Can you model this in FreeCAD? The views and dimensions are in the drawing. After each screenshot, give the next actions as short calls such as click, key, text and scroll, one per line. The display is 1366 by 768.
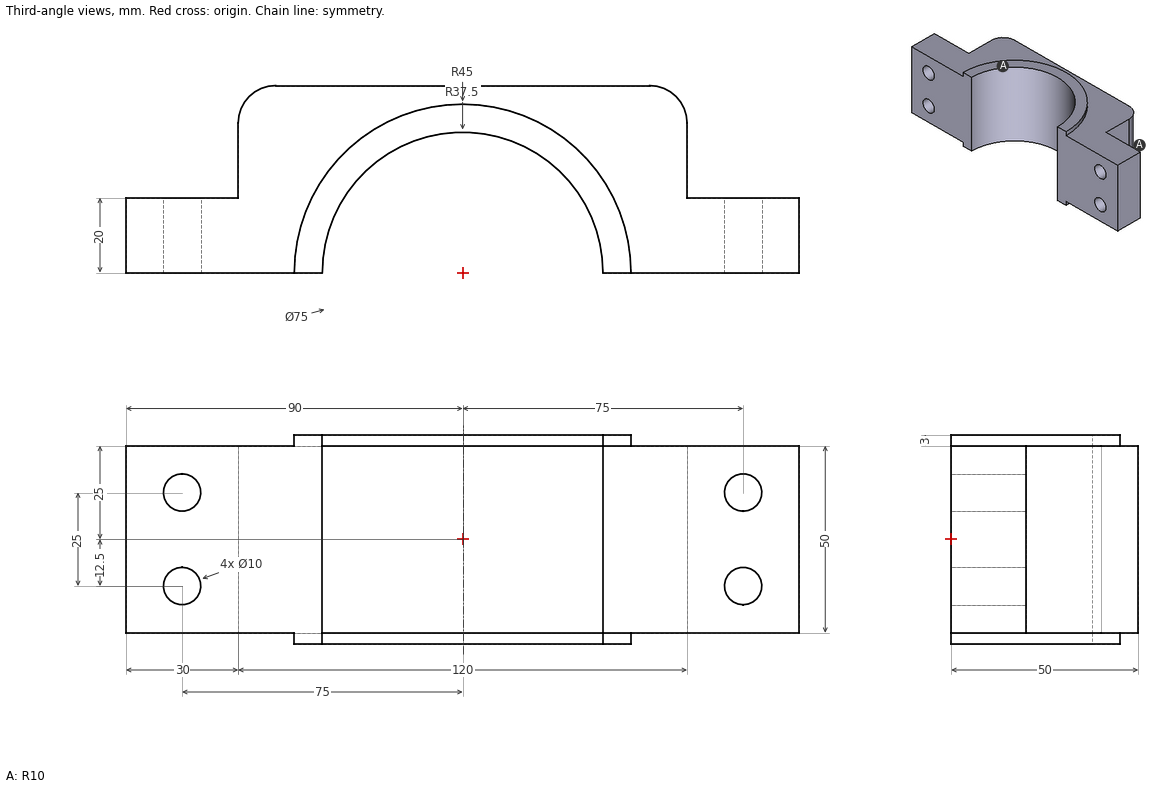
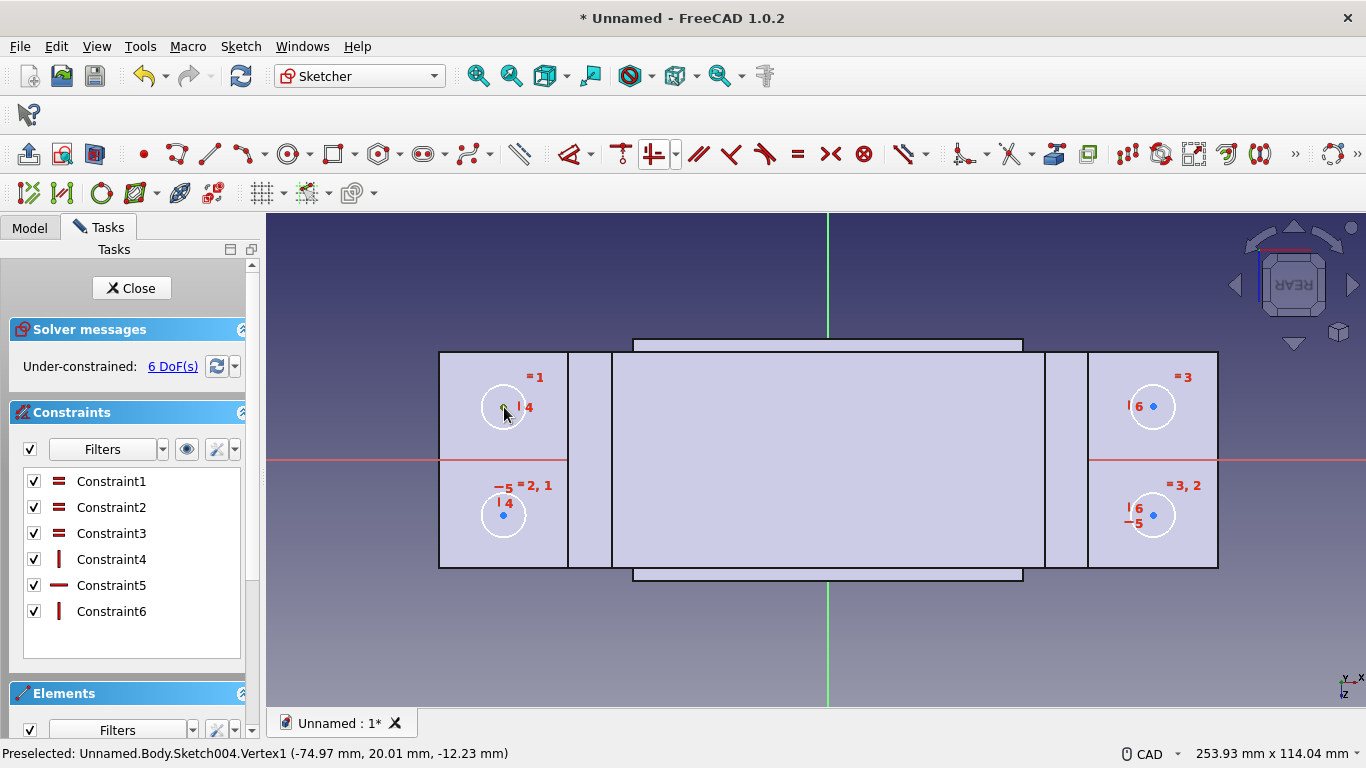
click(1153, 407)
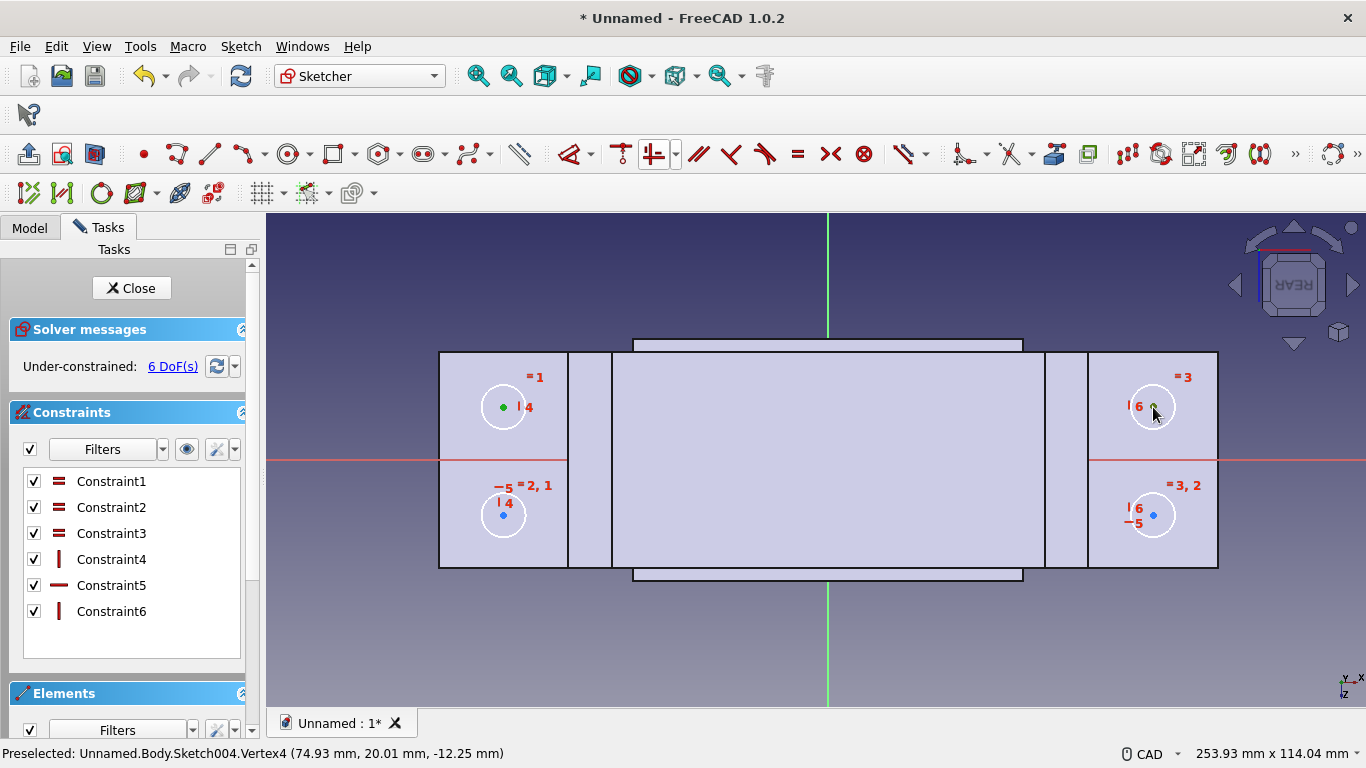
key(h)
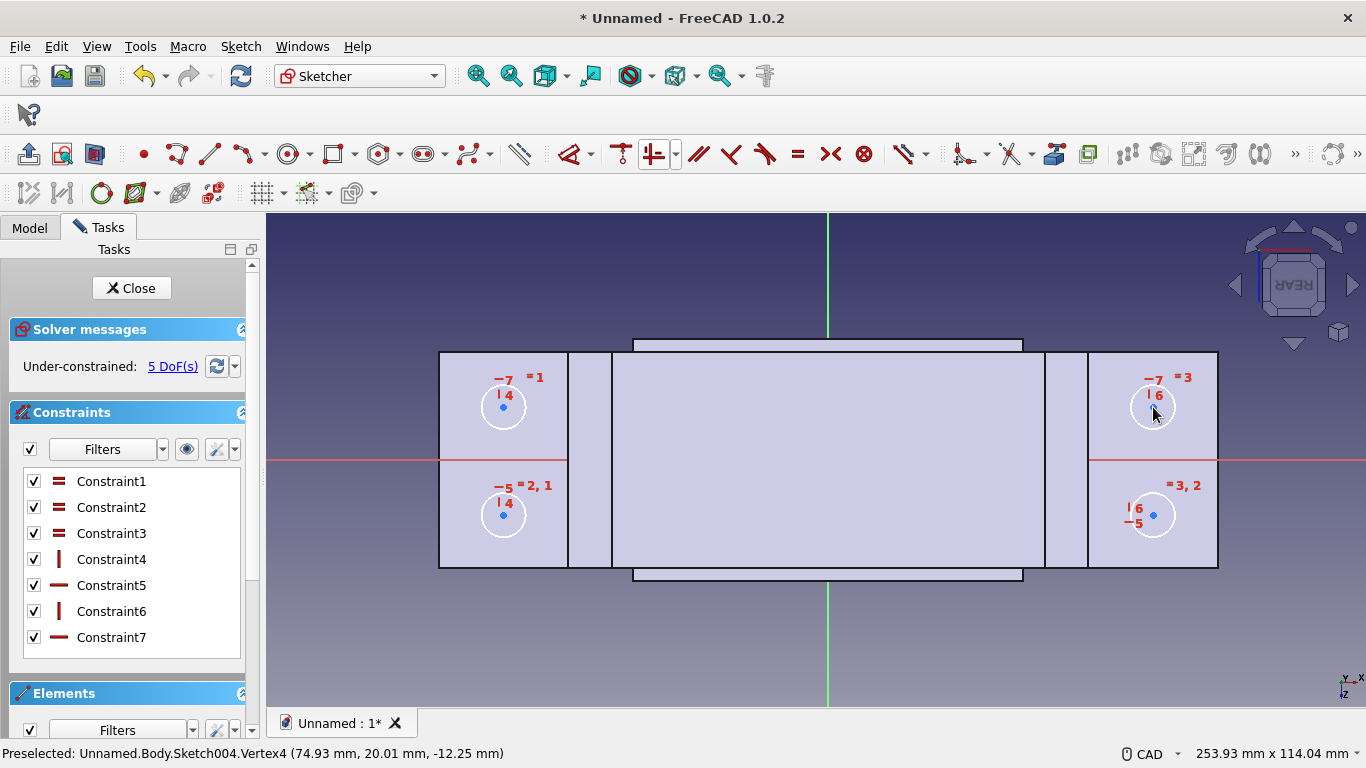
click(519, 391)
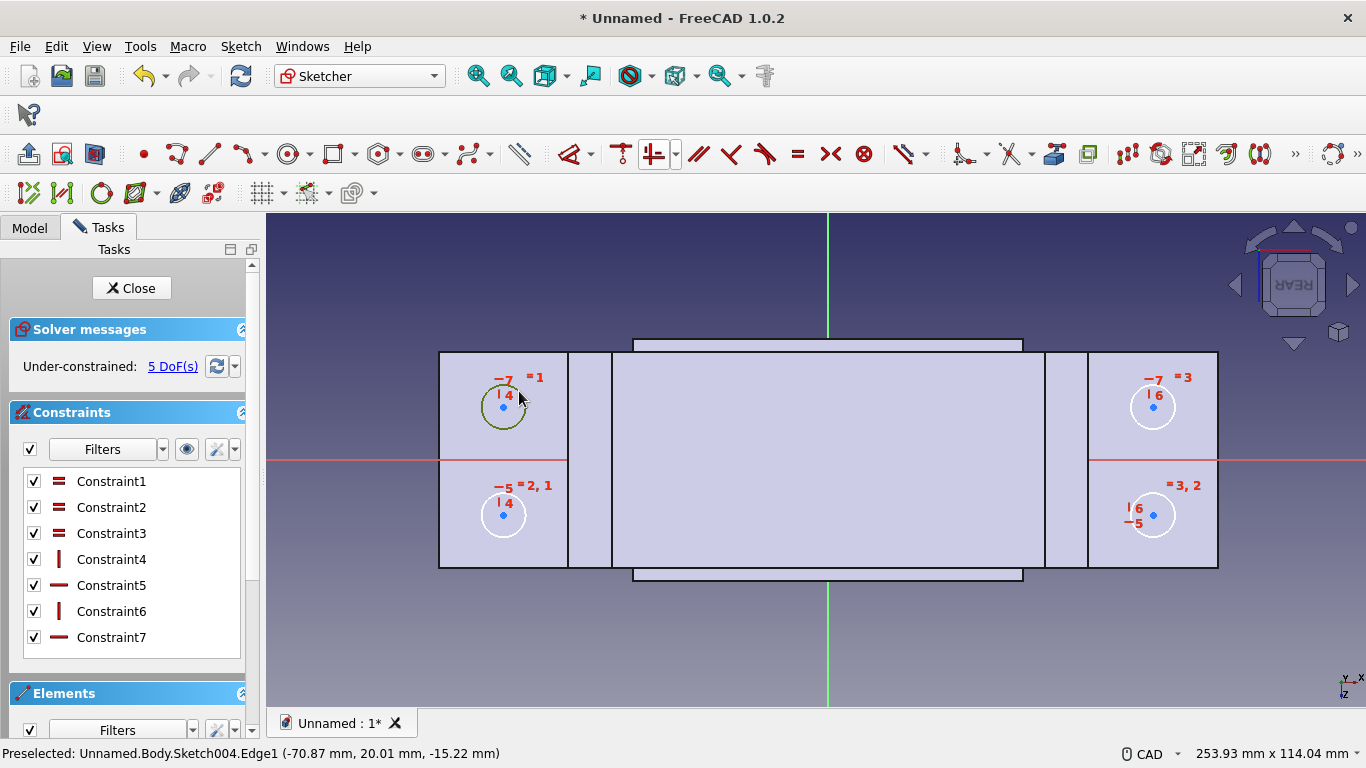
key(k)
key(o)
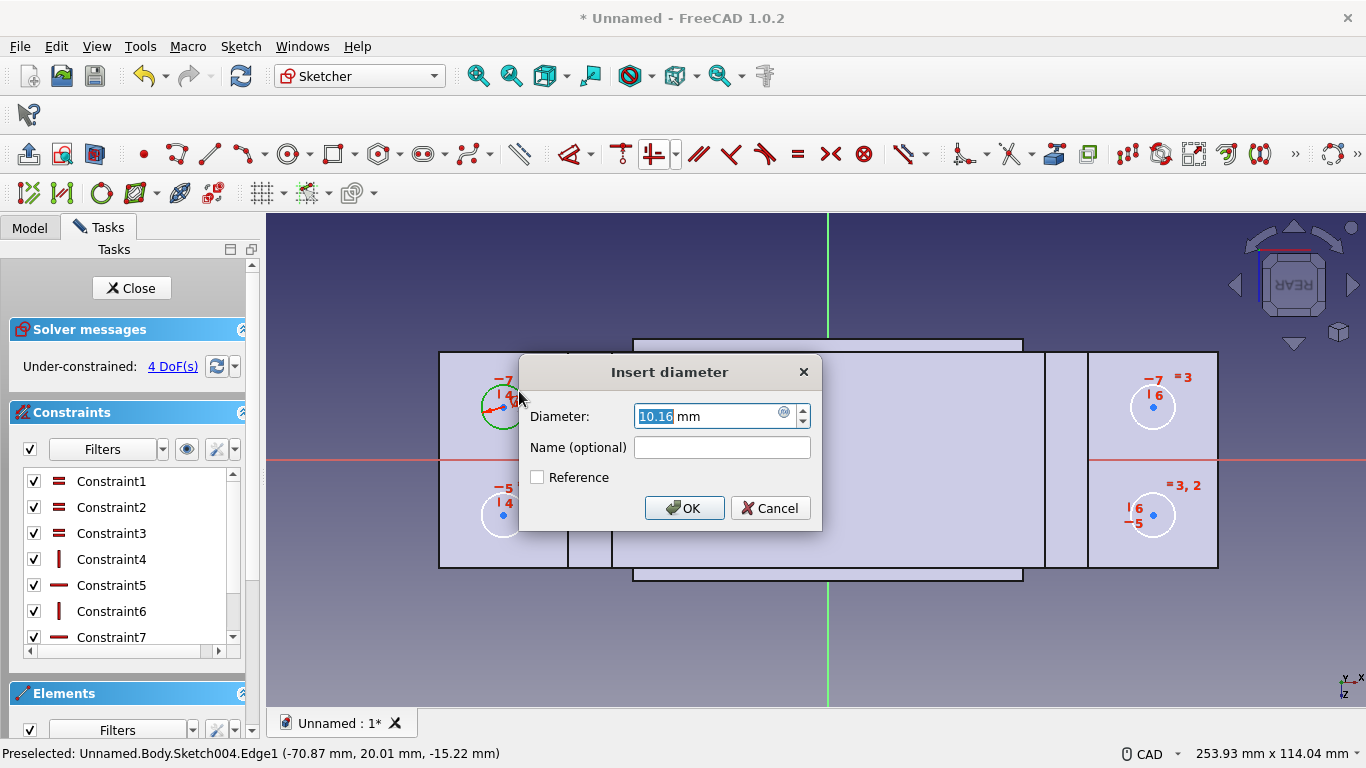
text(10)
key(Return)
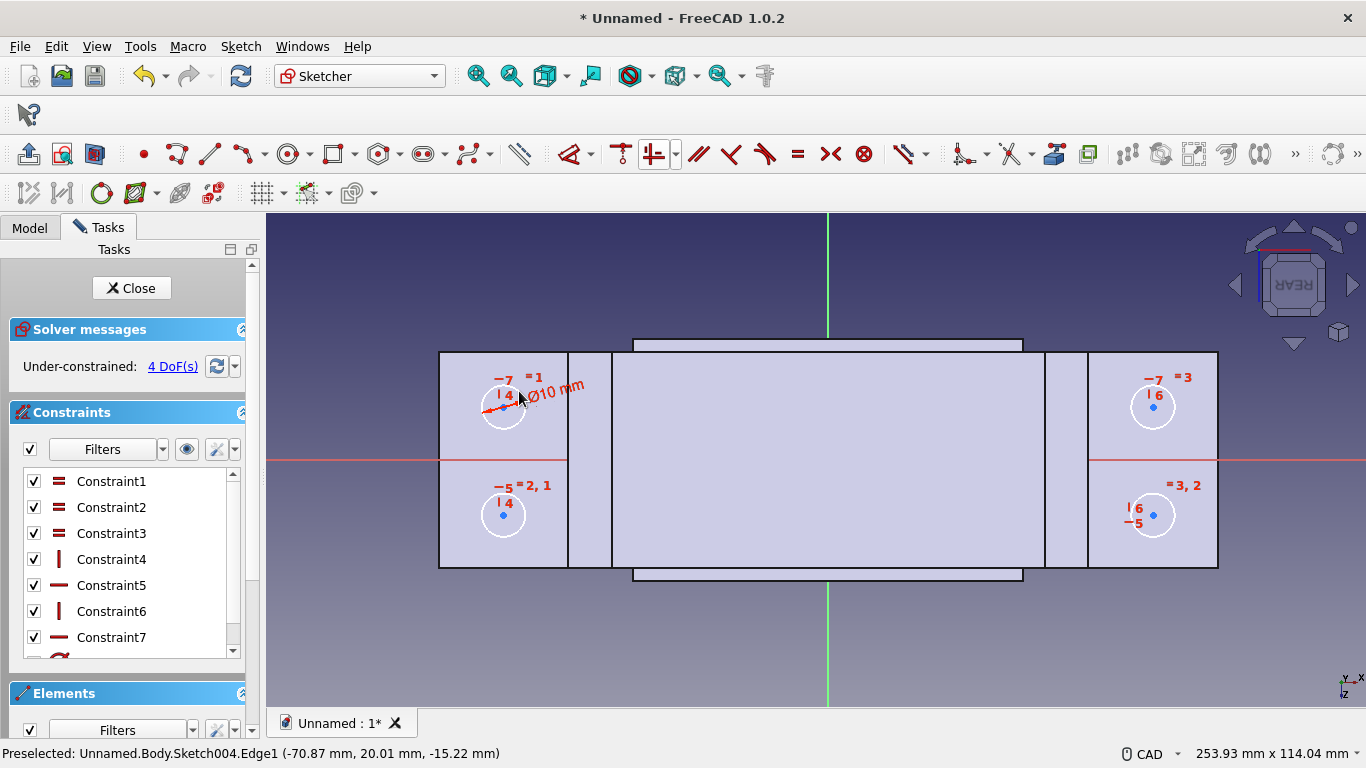
click(504, 407)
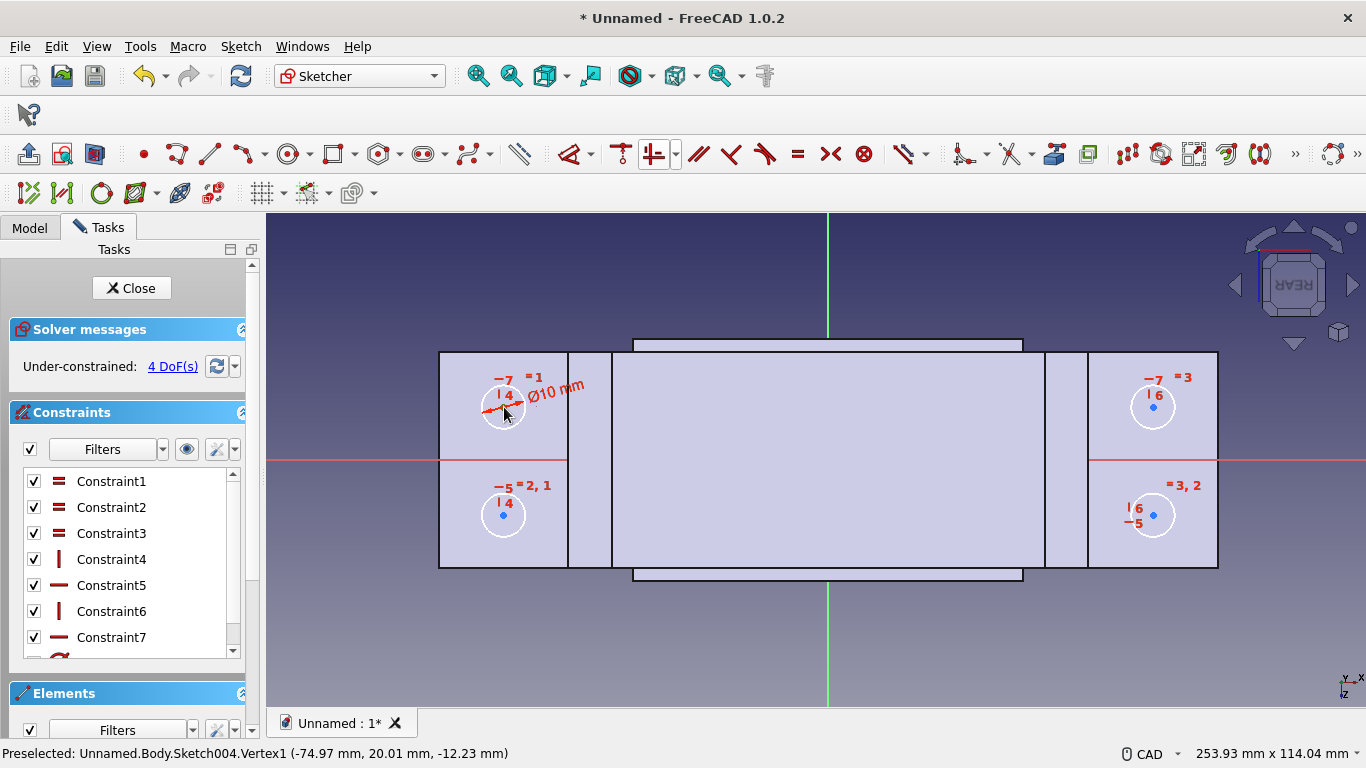
click(590, 154)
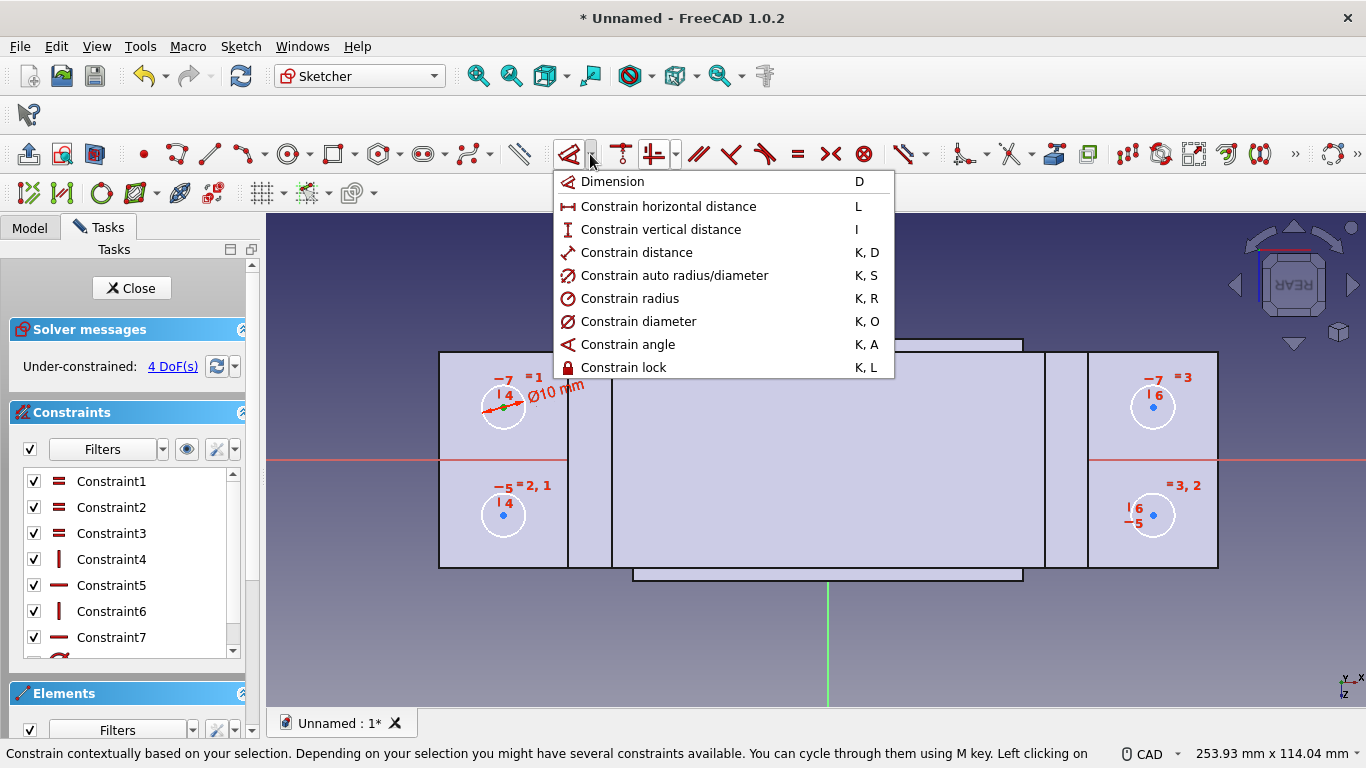
click(724, 206)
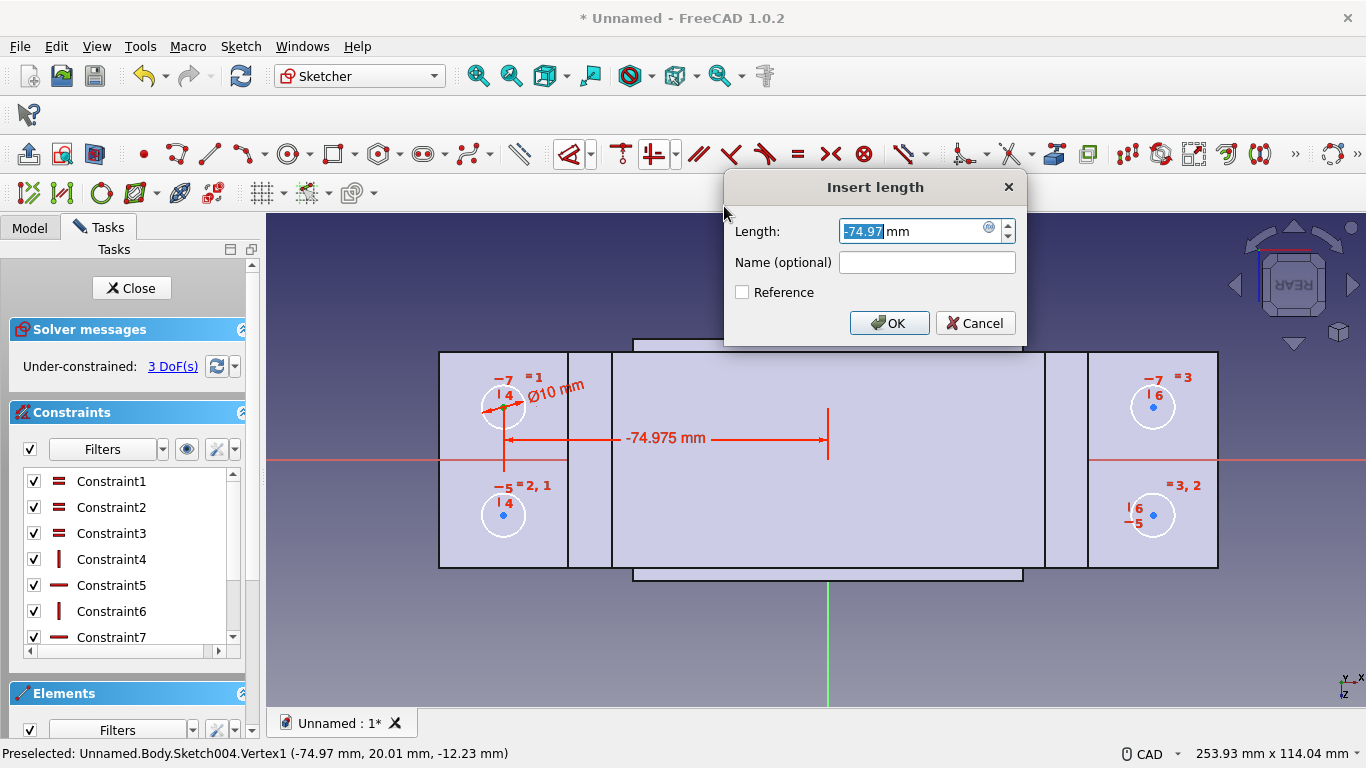
text(-75)
key(Return)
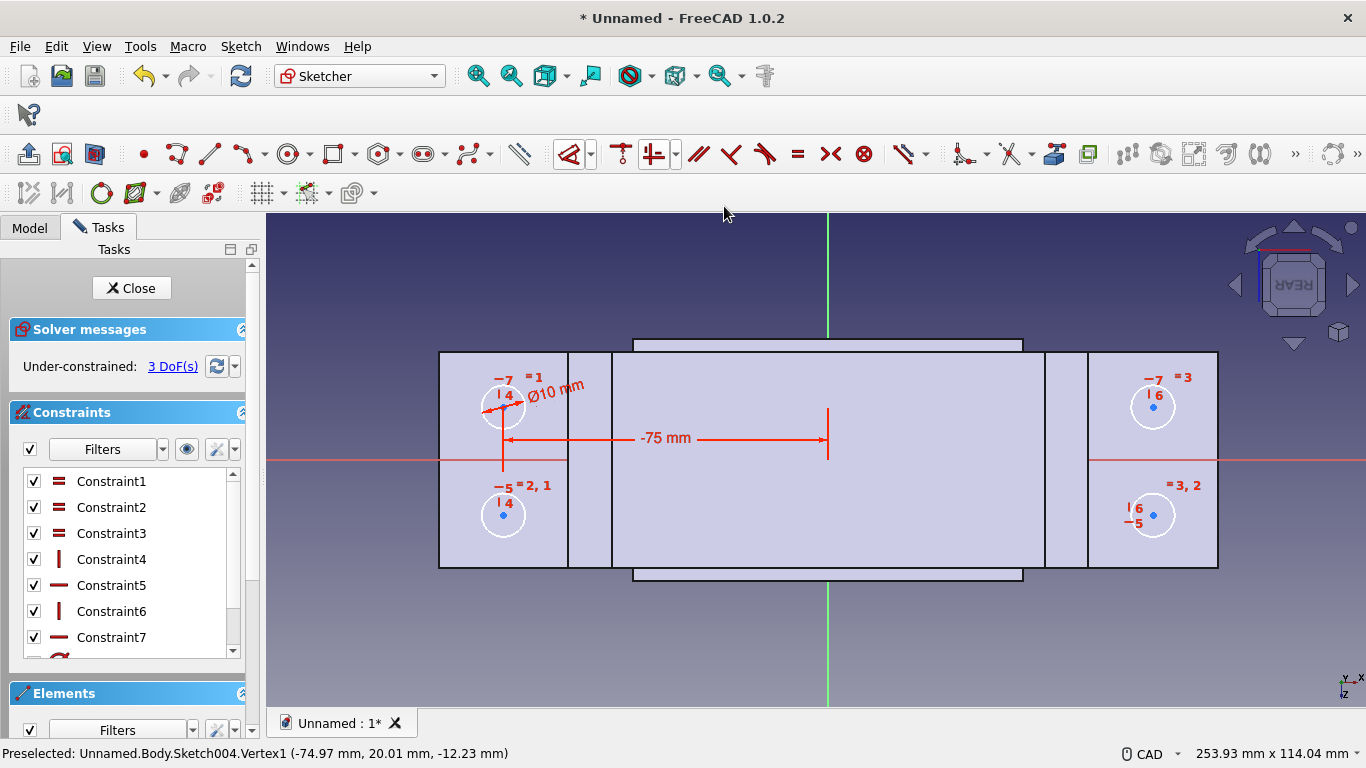
click(1153, 515)